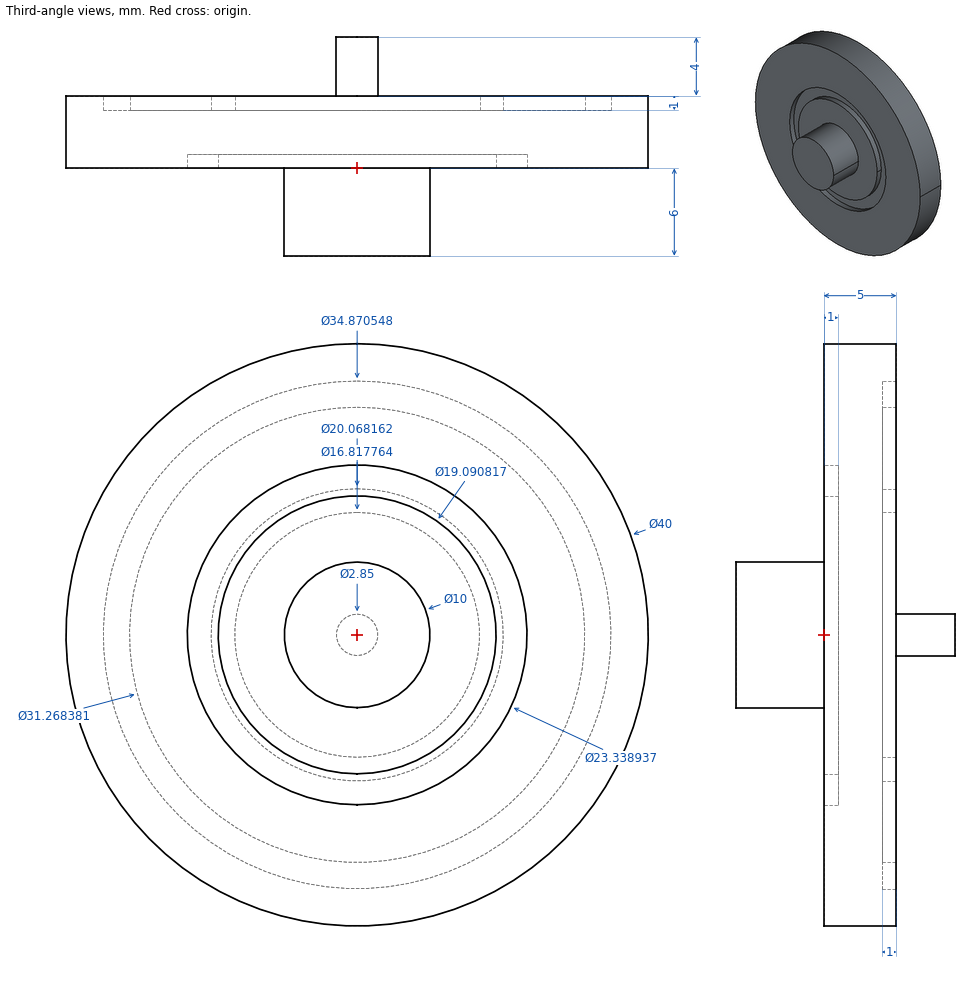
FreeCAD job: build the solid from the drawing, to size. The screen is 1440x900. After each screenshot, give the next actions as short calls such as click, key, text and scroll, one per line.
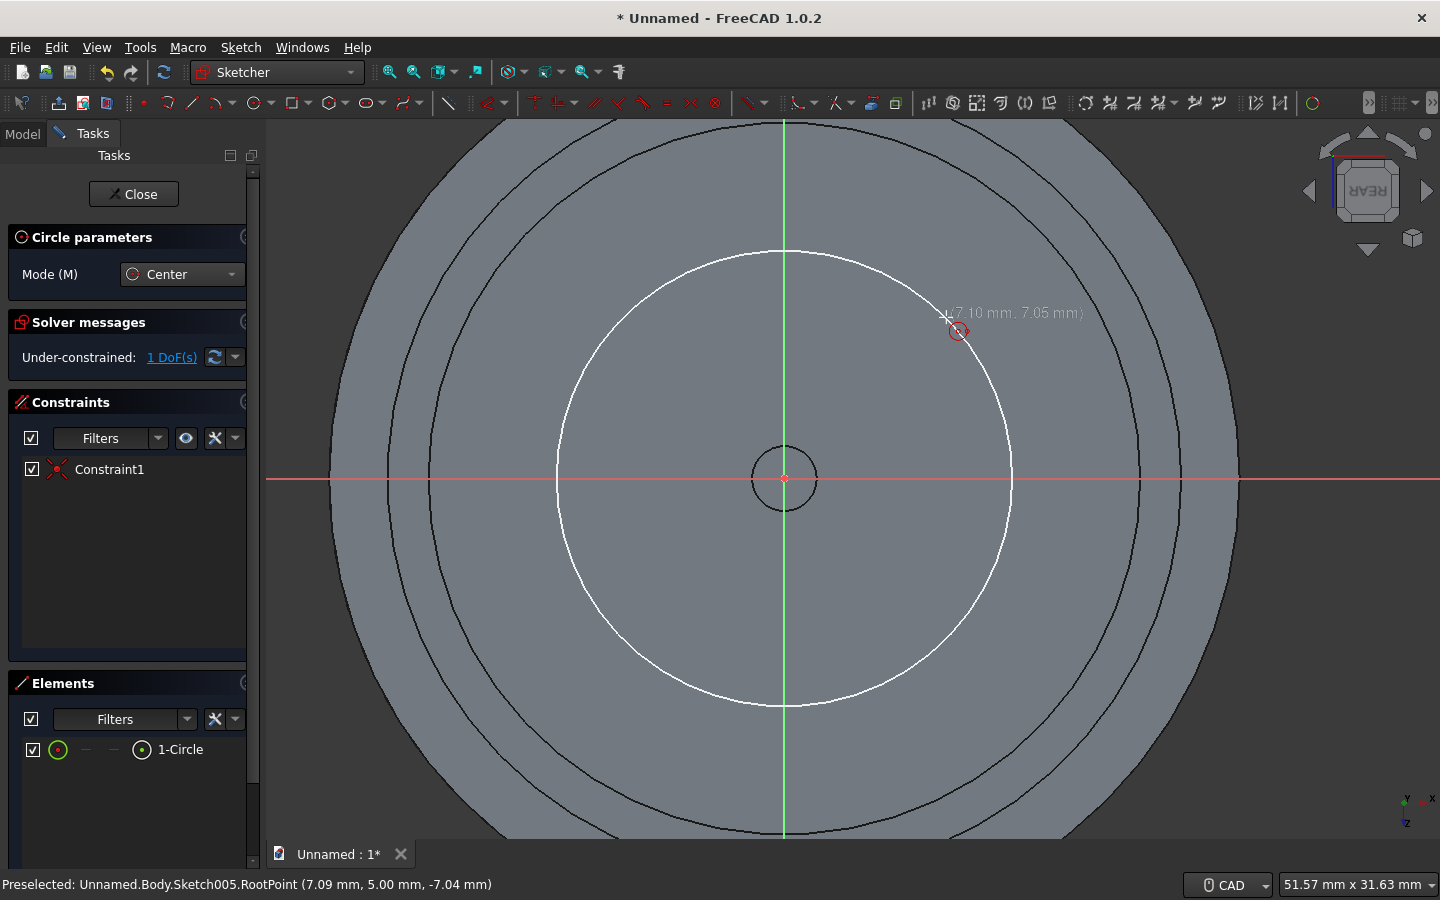
click(784, 479)
click(920, 343)
key(Escape)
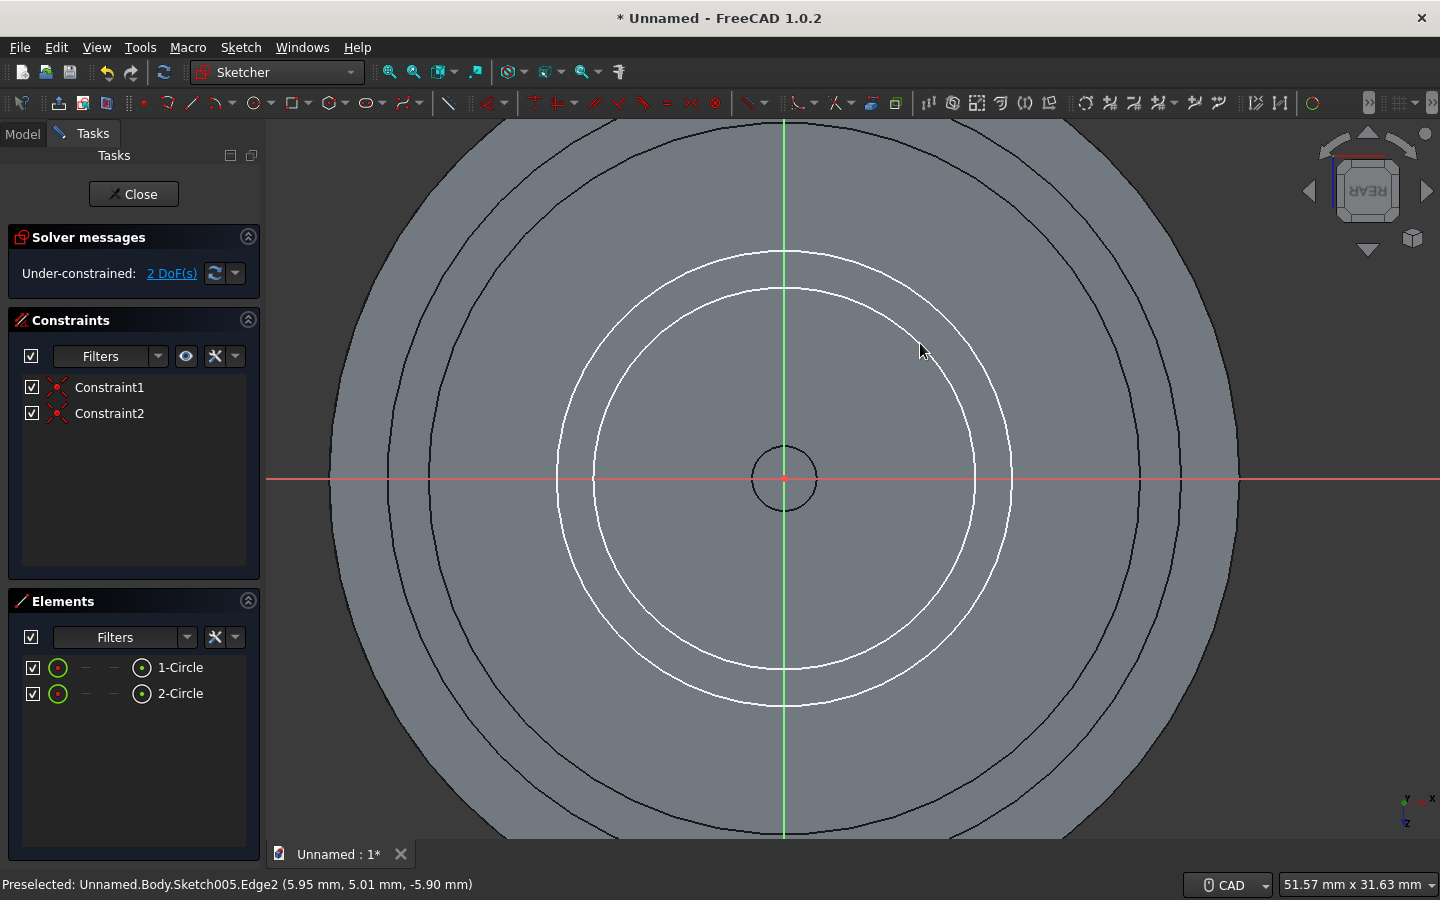
key(d)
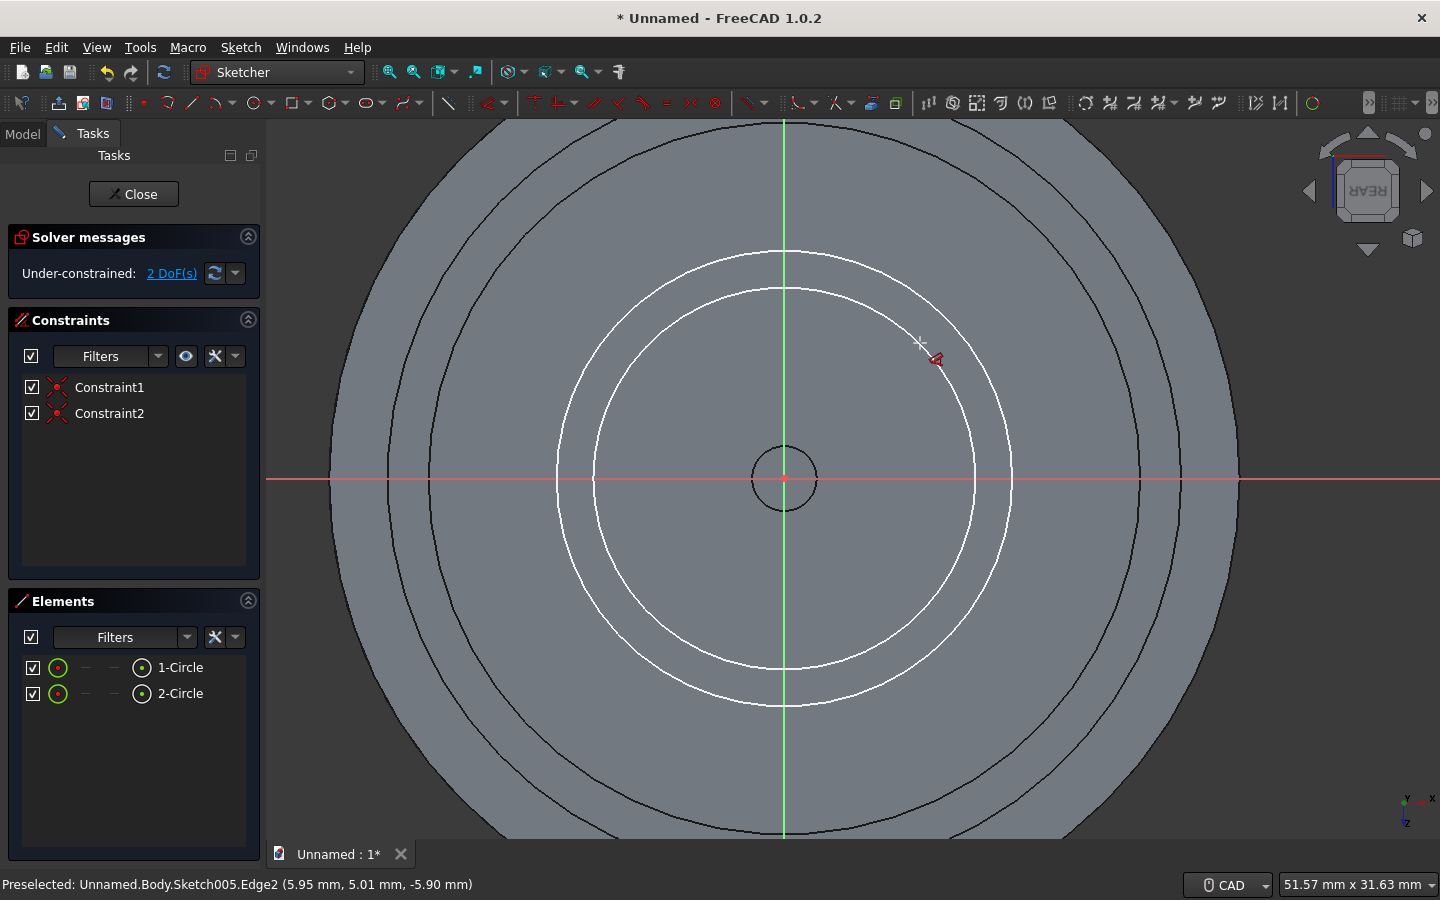
click(945, 317)
click(968, 294)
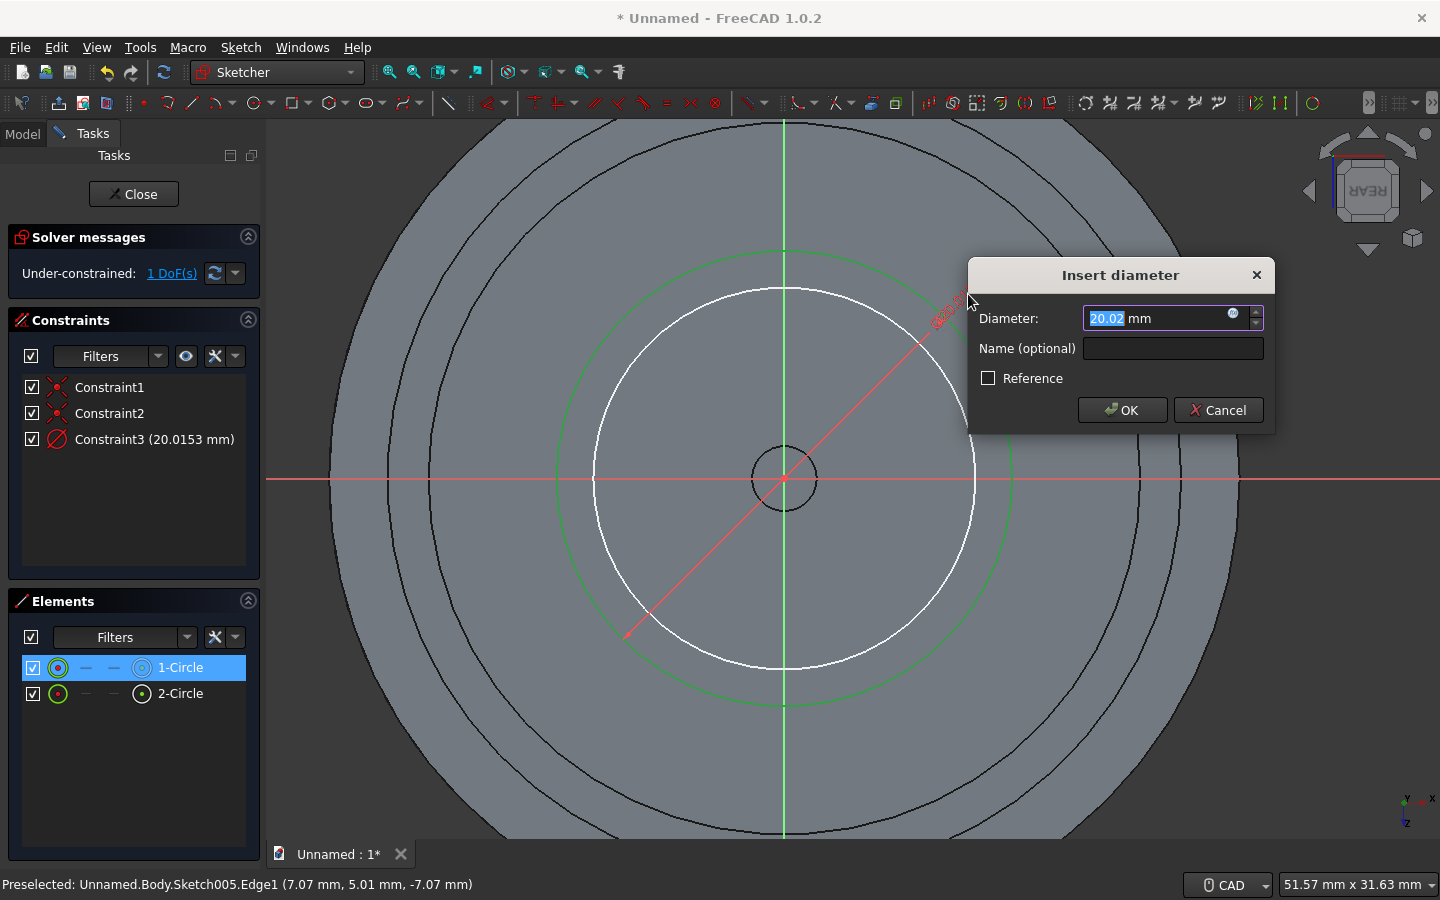
text(20.068162)
key(Return)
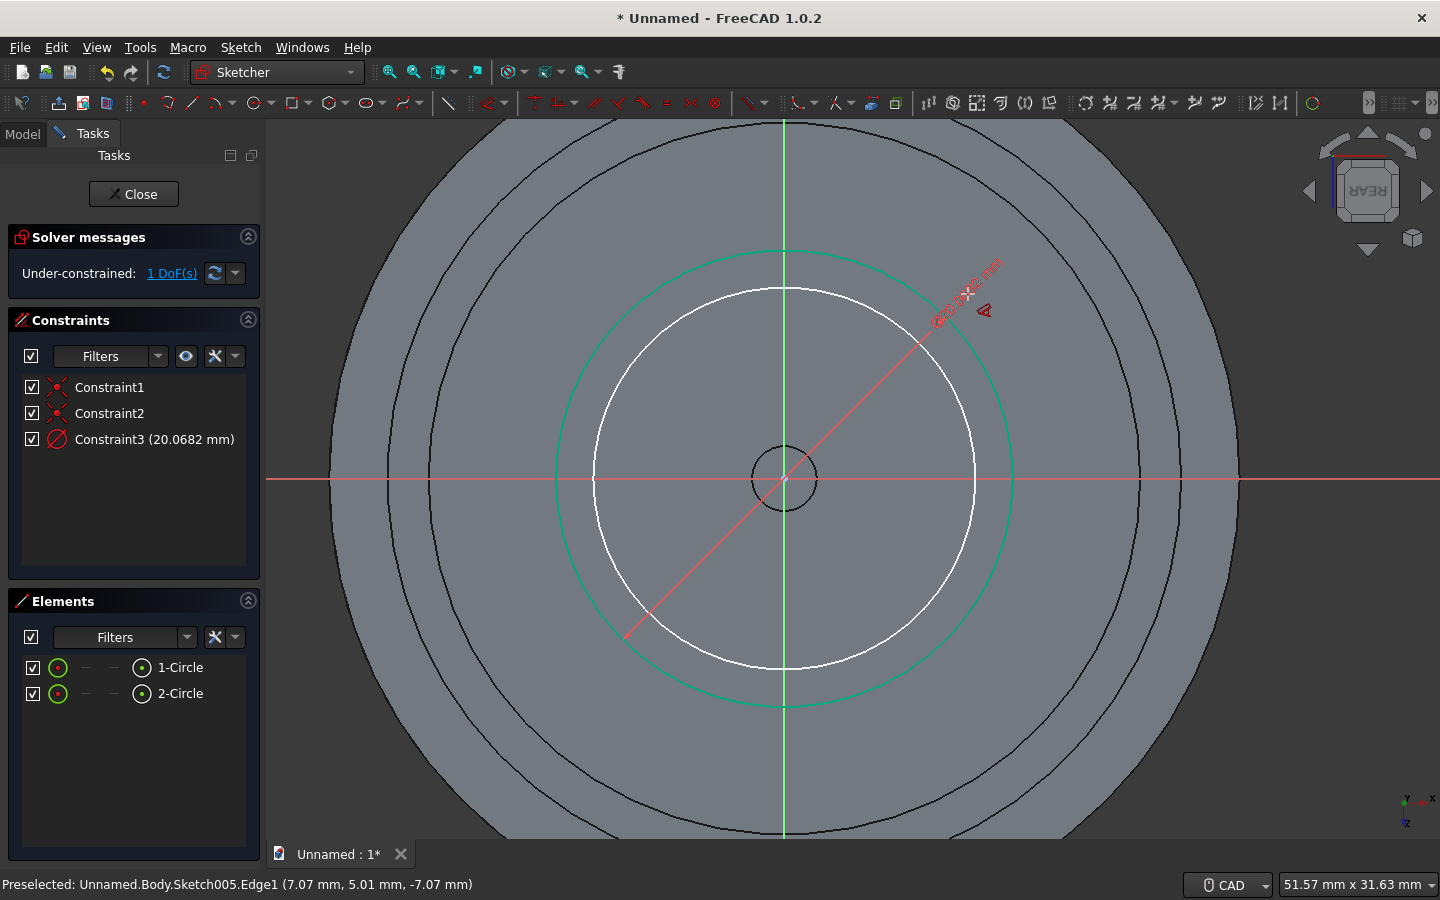
click(919, 343)
click(1020, 408)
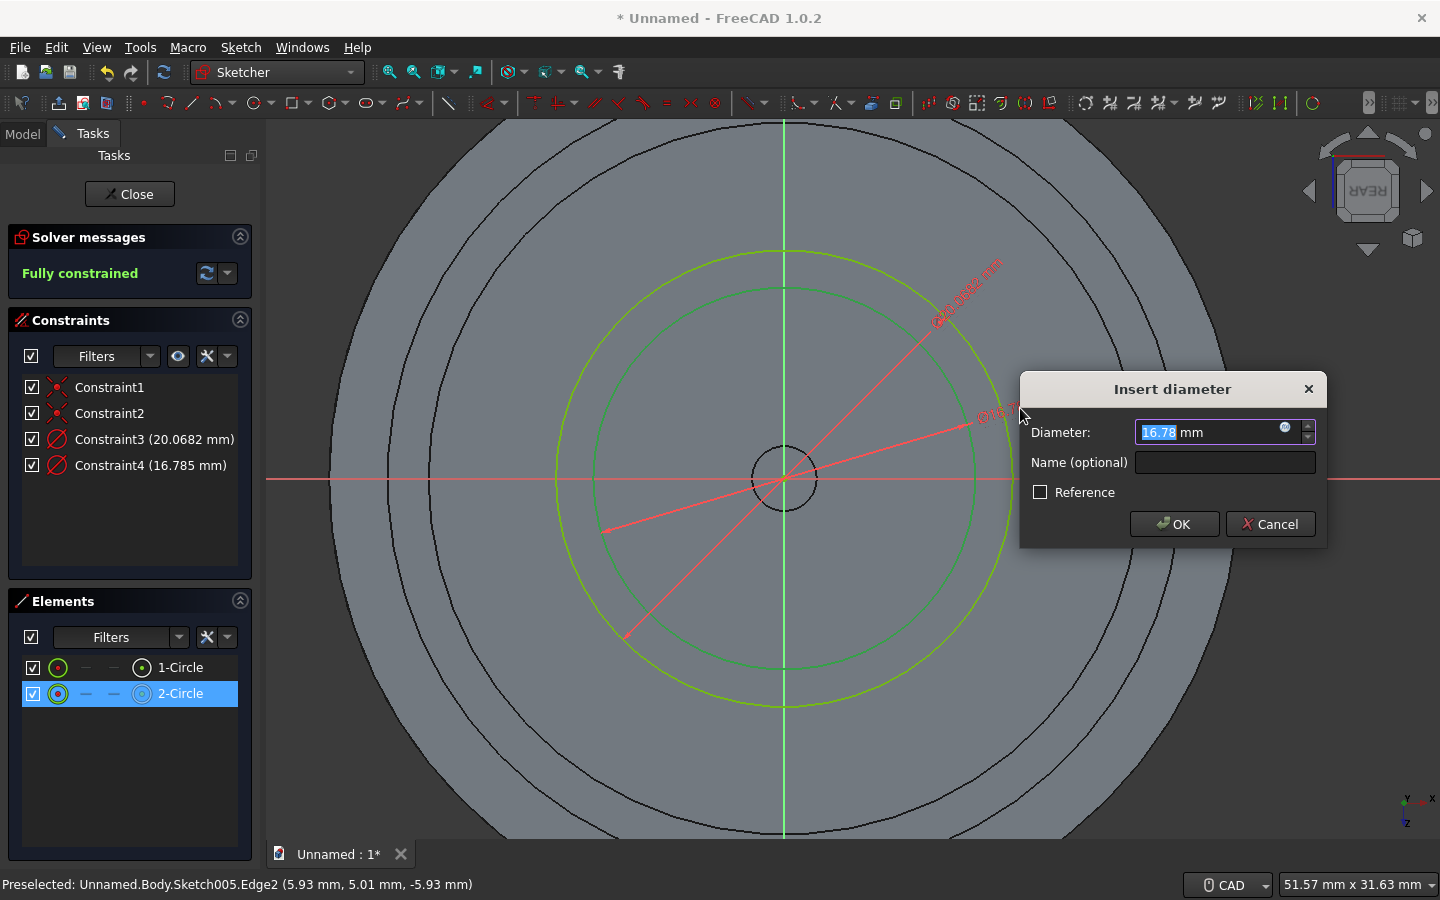
text(16.817764)
key(Return)
key(Escape)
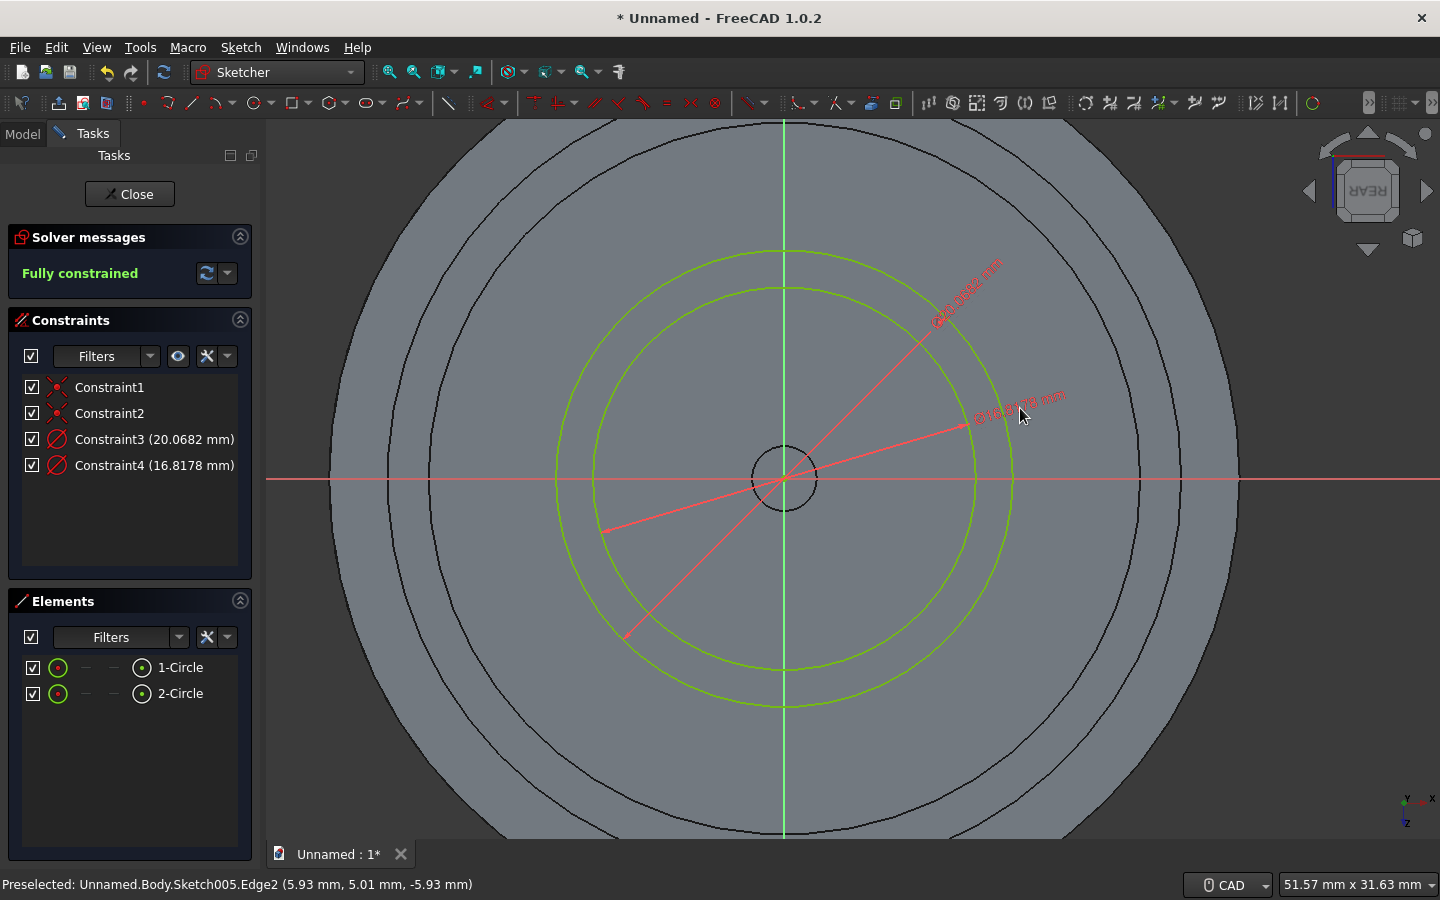
click(130, 194)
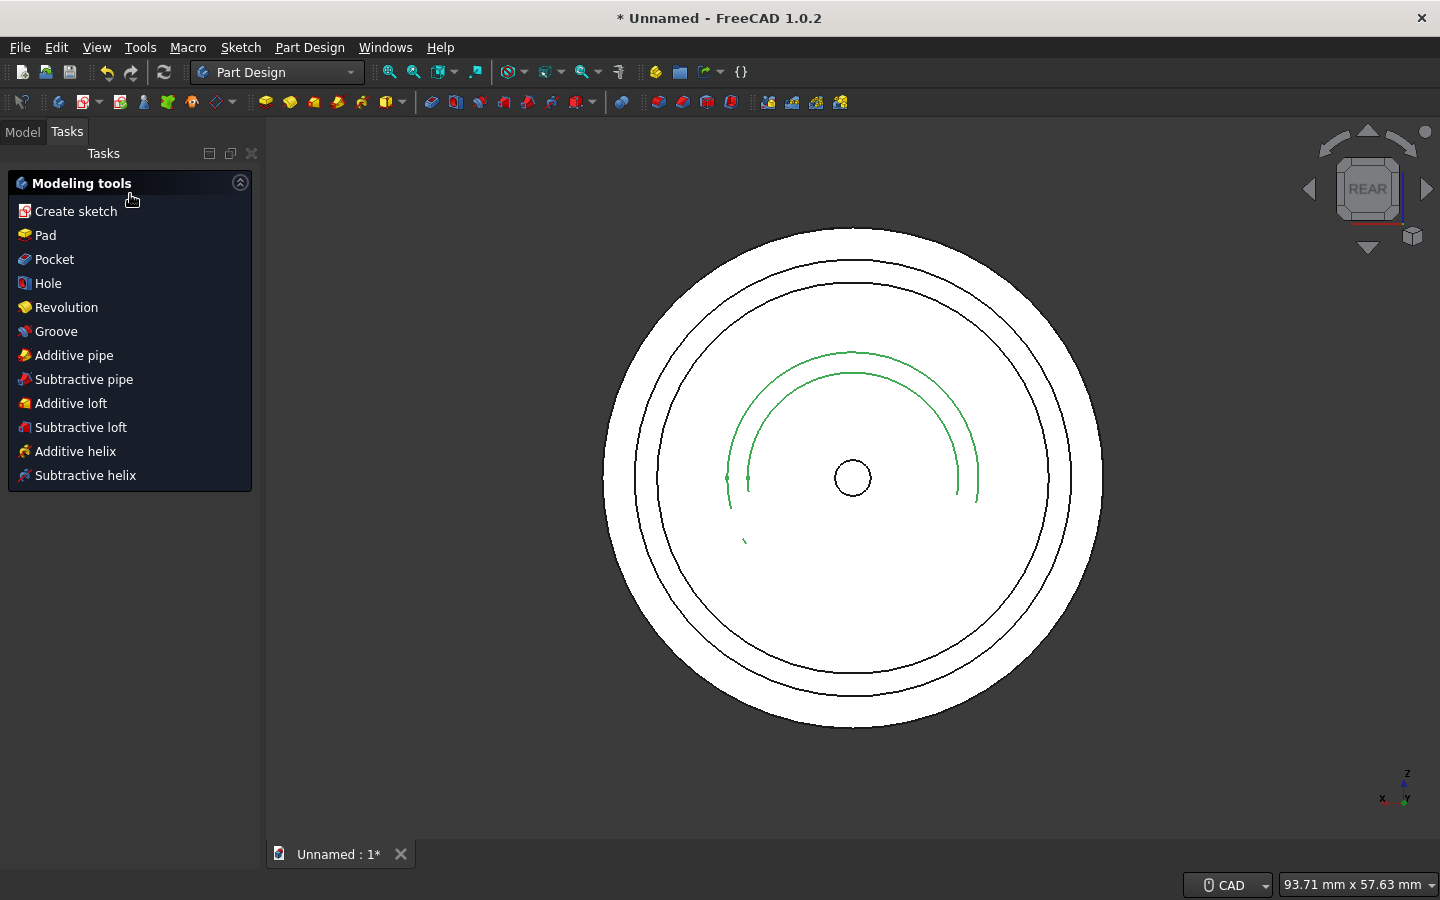
click(432, 102)